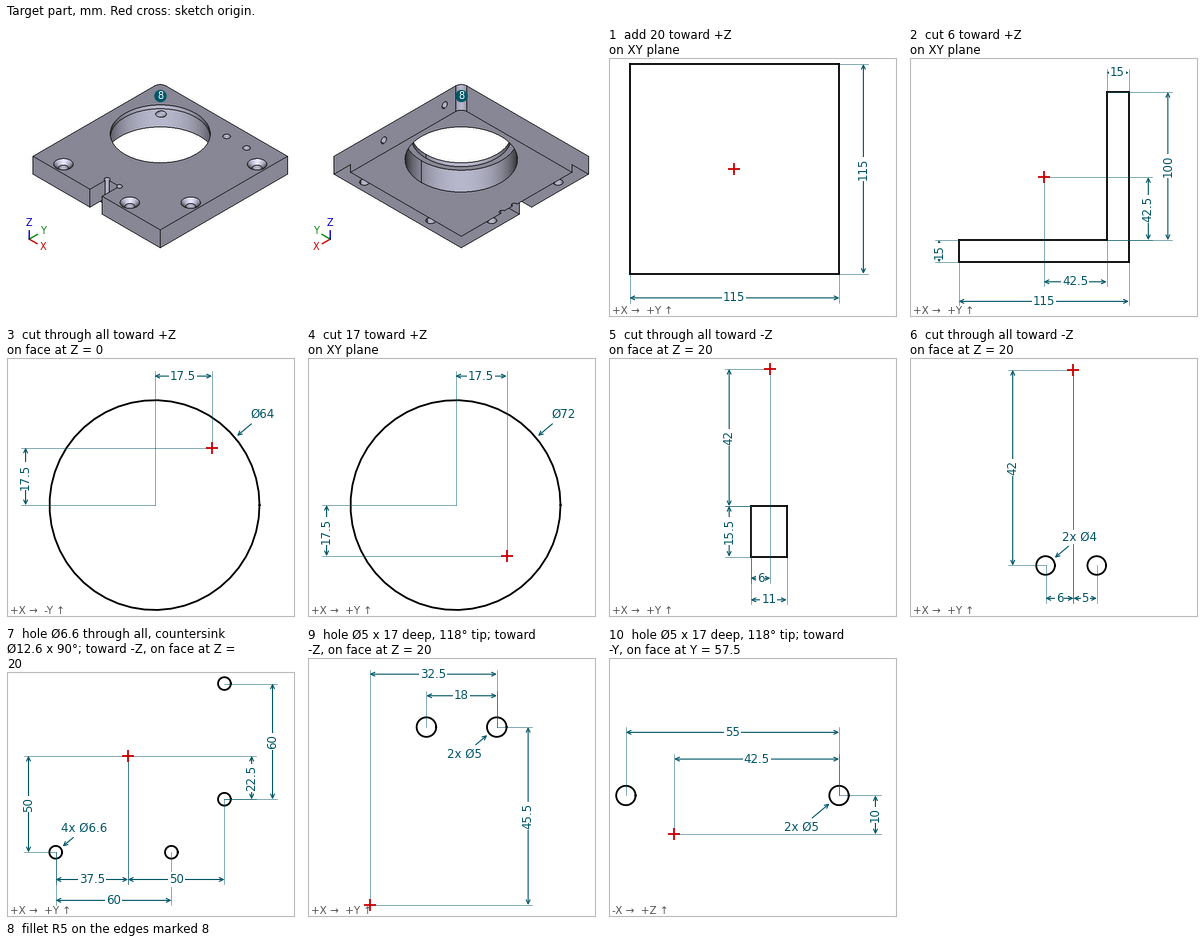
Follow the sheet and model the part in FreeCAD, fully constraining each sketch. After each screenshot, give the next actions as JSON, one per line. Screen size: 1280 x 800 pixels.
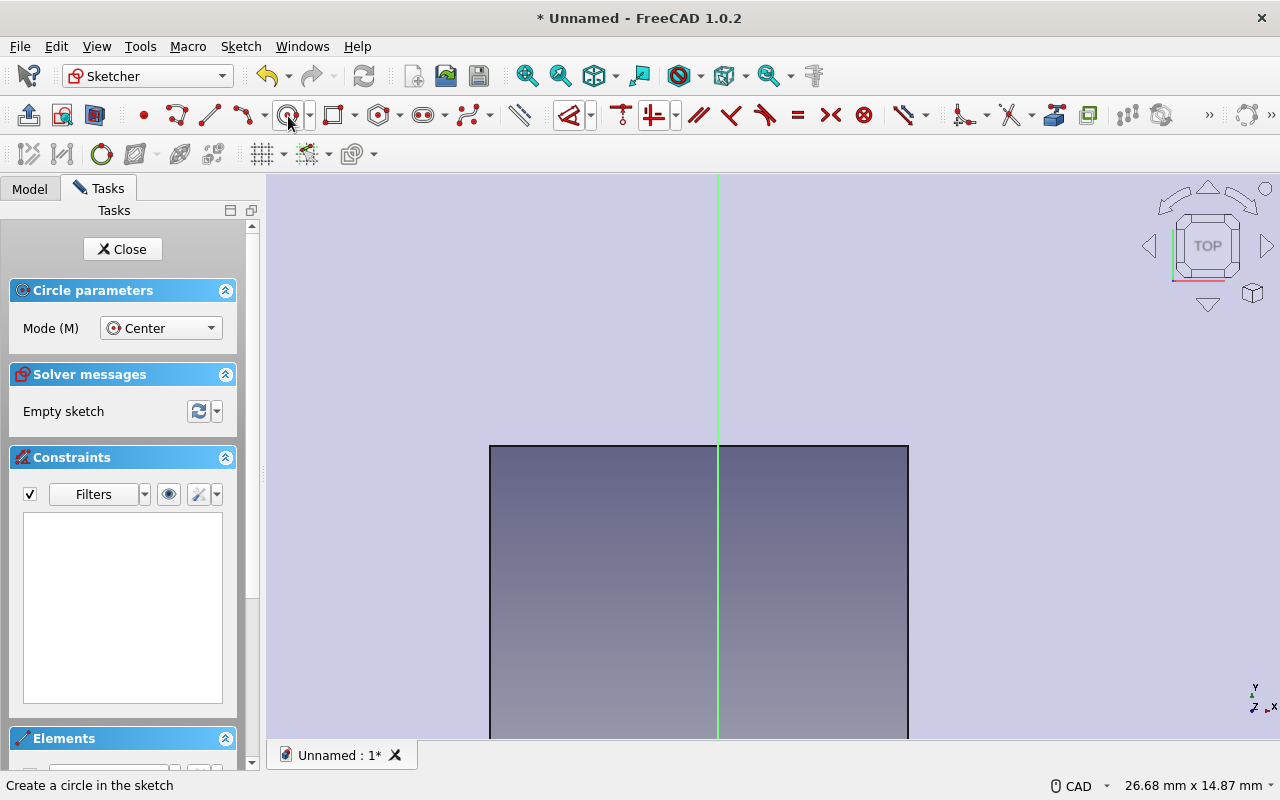
{"action": "left_click", "coordinate": [490, 446]}
{"action": "left_click", "coordinate": [544, 393]}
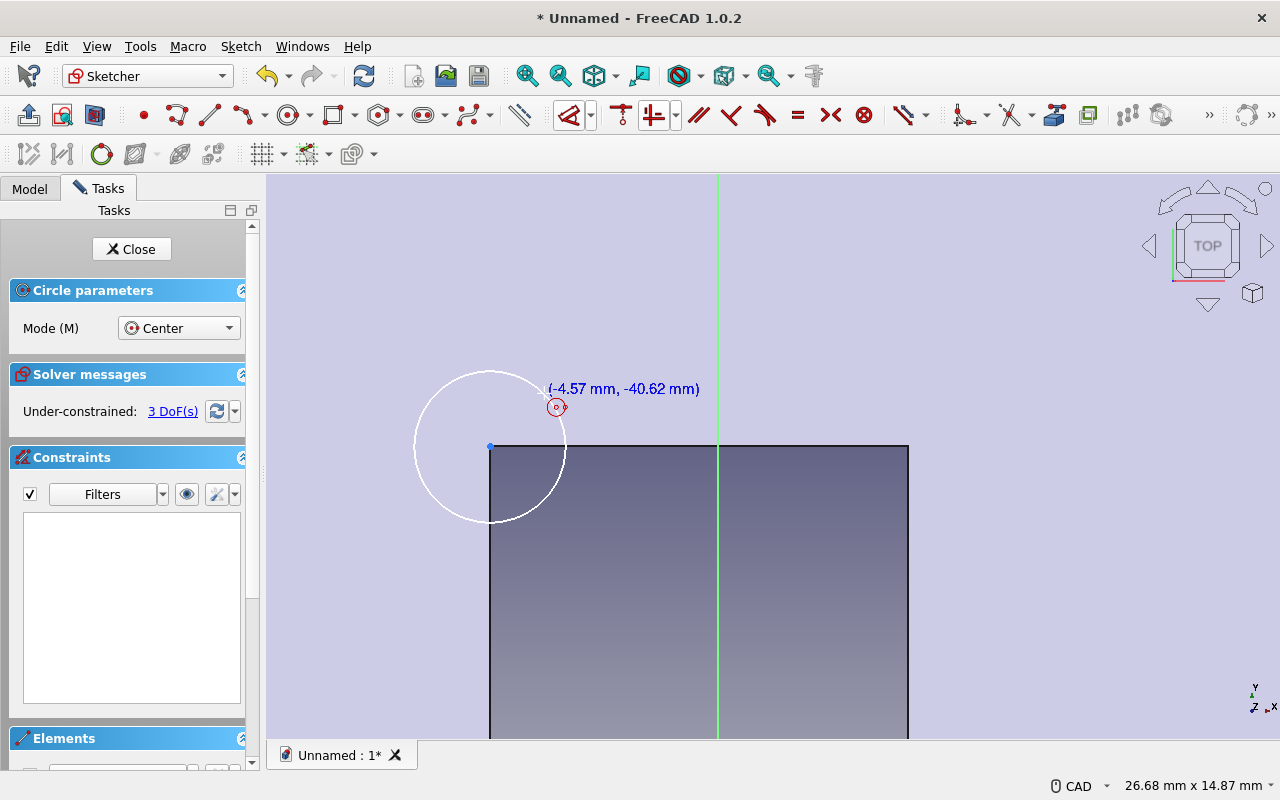
{"action": "left_click", "coordinate": [908, 446]}
{"action": "left_click", "coordinate": [962, 393]}
{"action": "key", "text": "Escape"}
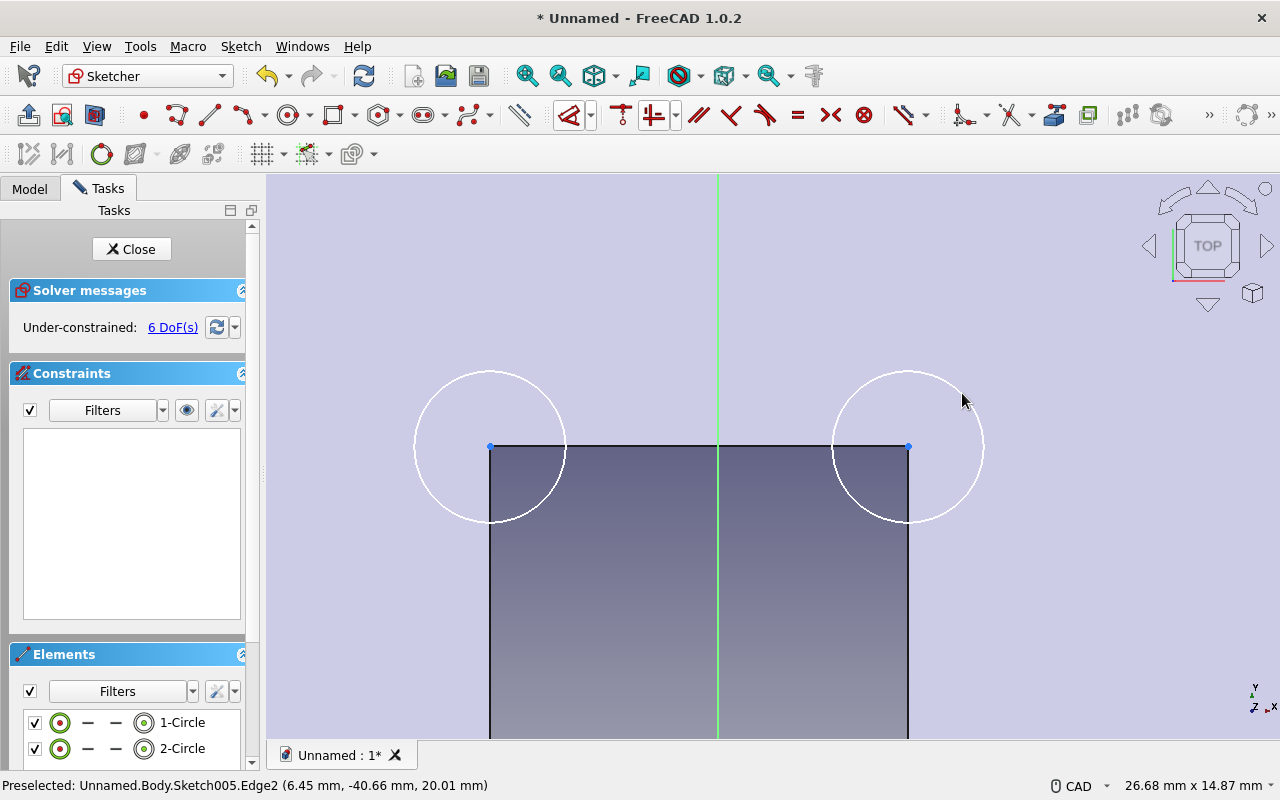
{"action": "left_click", "coordinate": [543, 393]}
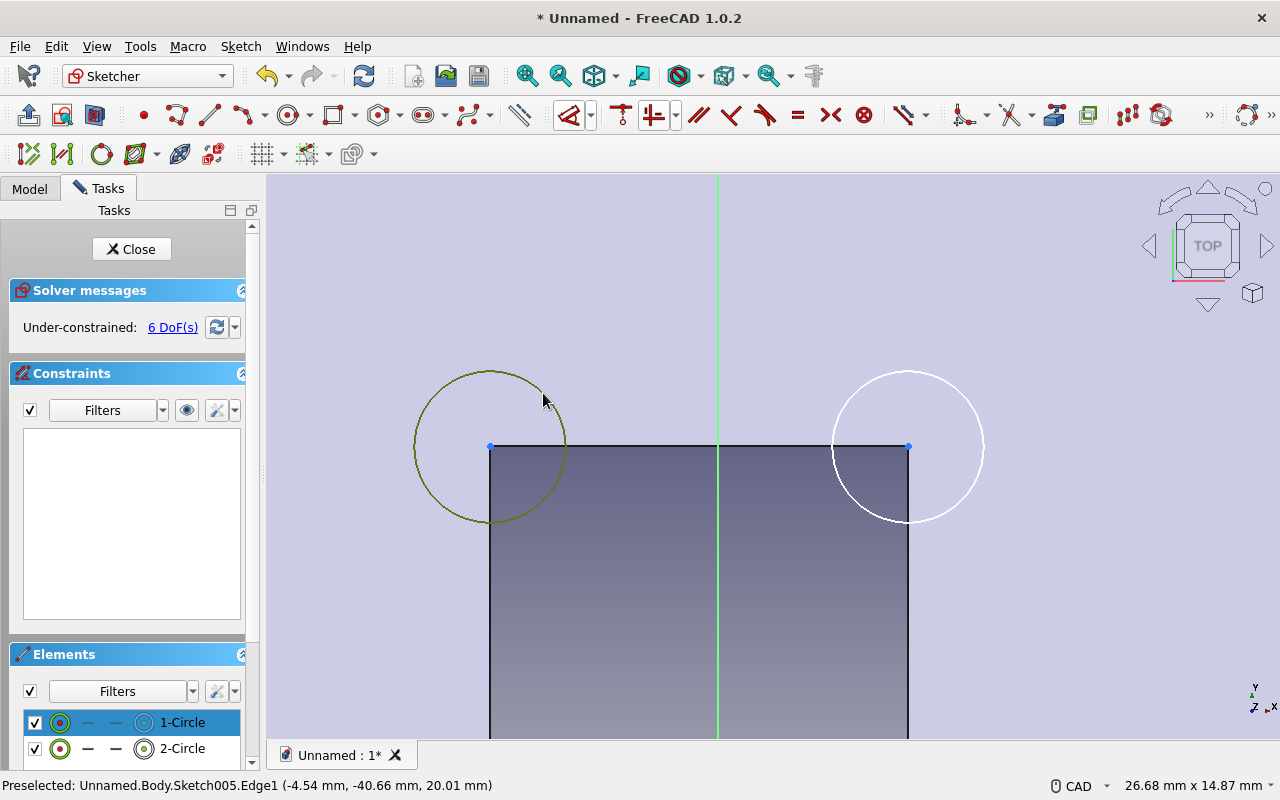
{"action": "left_click", "coordinate": [961, 393]}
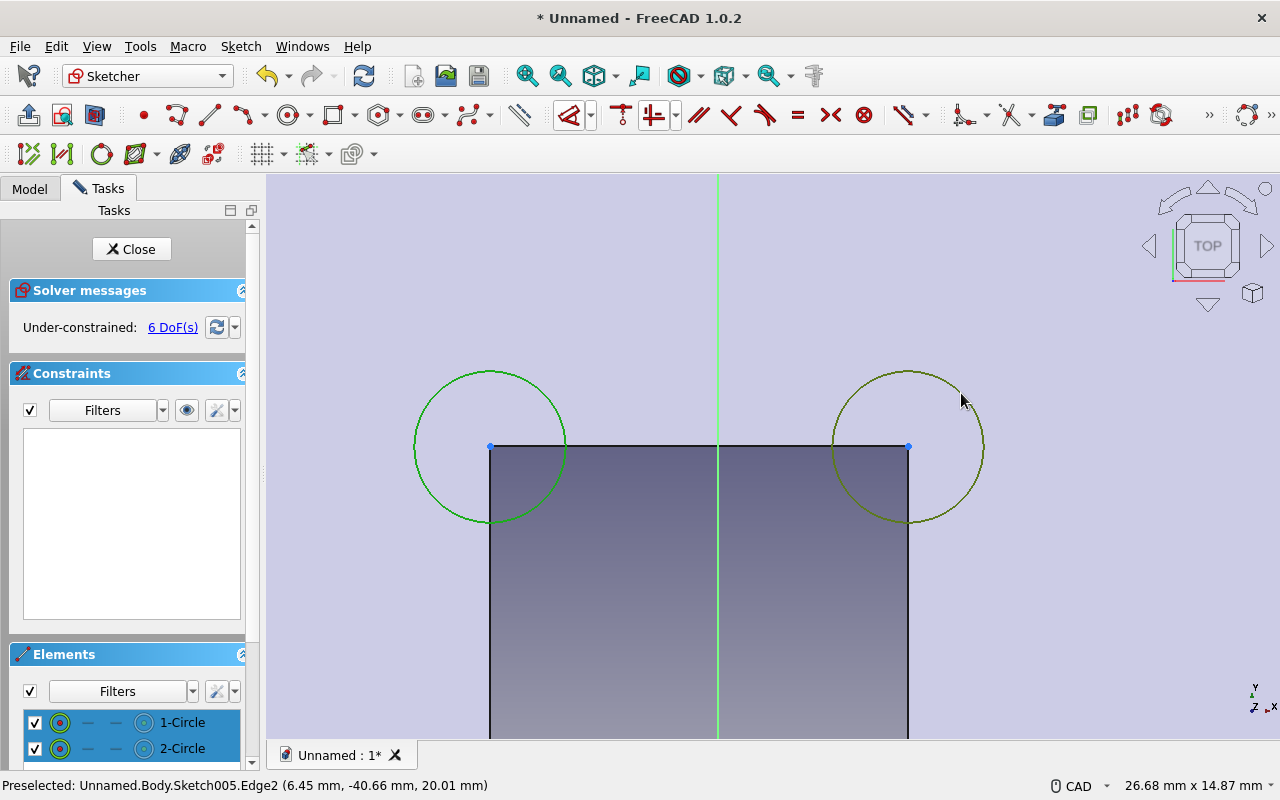
{"action": "key", "text": "e"}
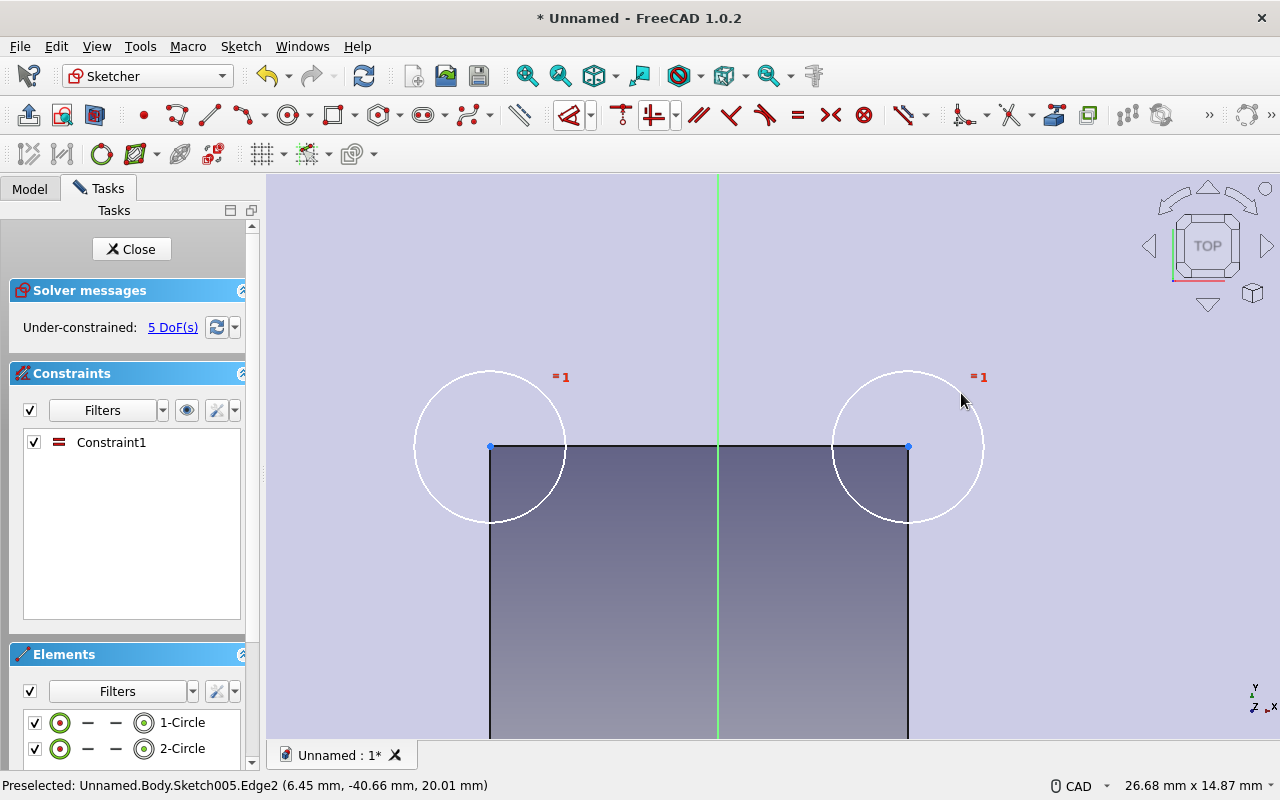
{"action": "left_click", "coordinate": [490, 447]}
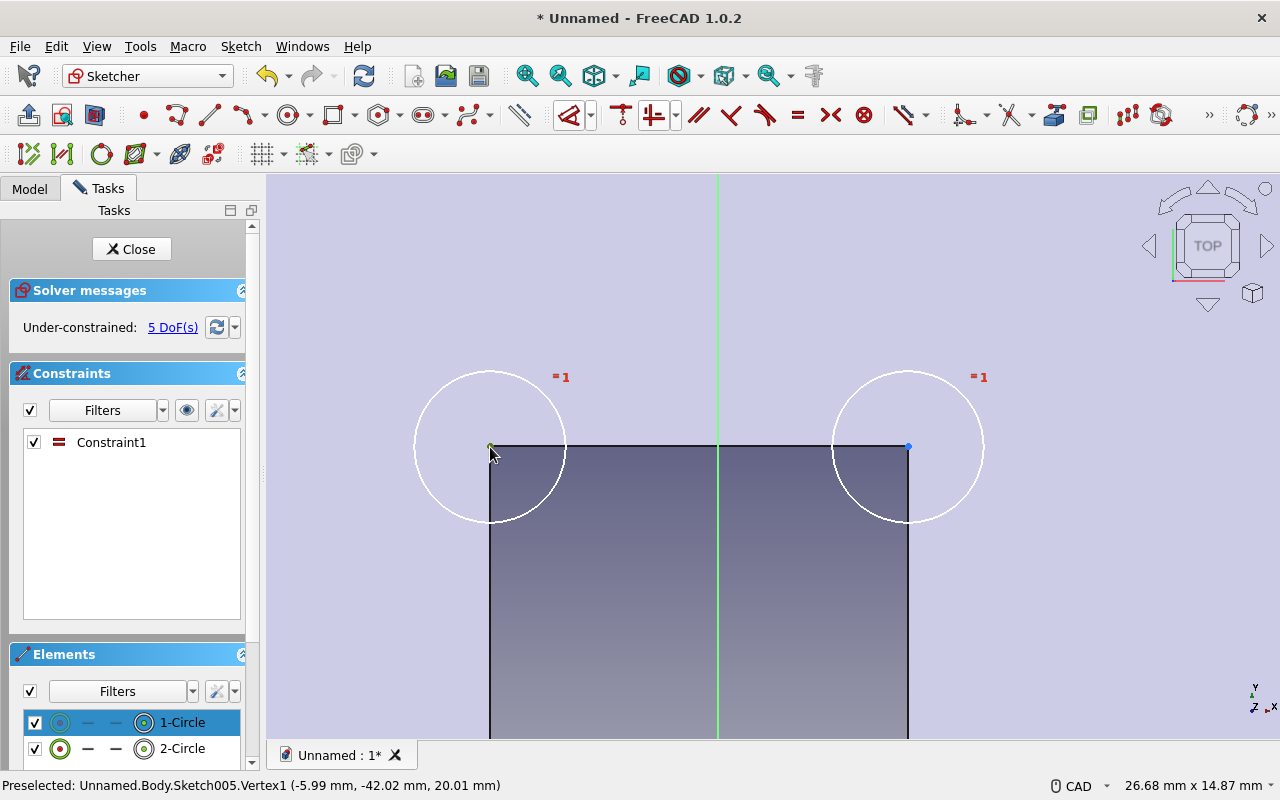
{"action": "left_click", "coordinate": [908, 447]}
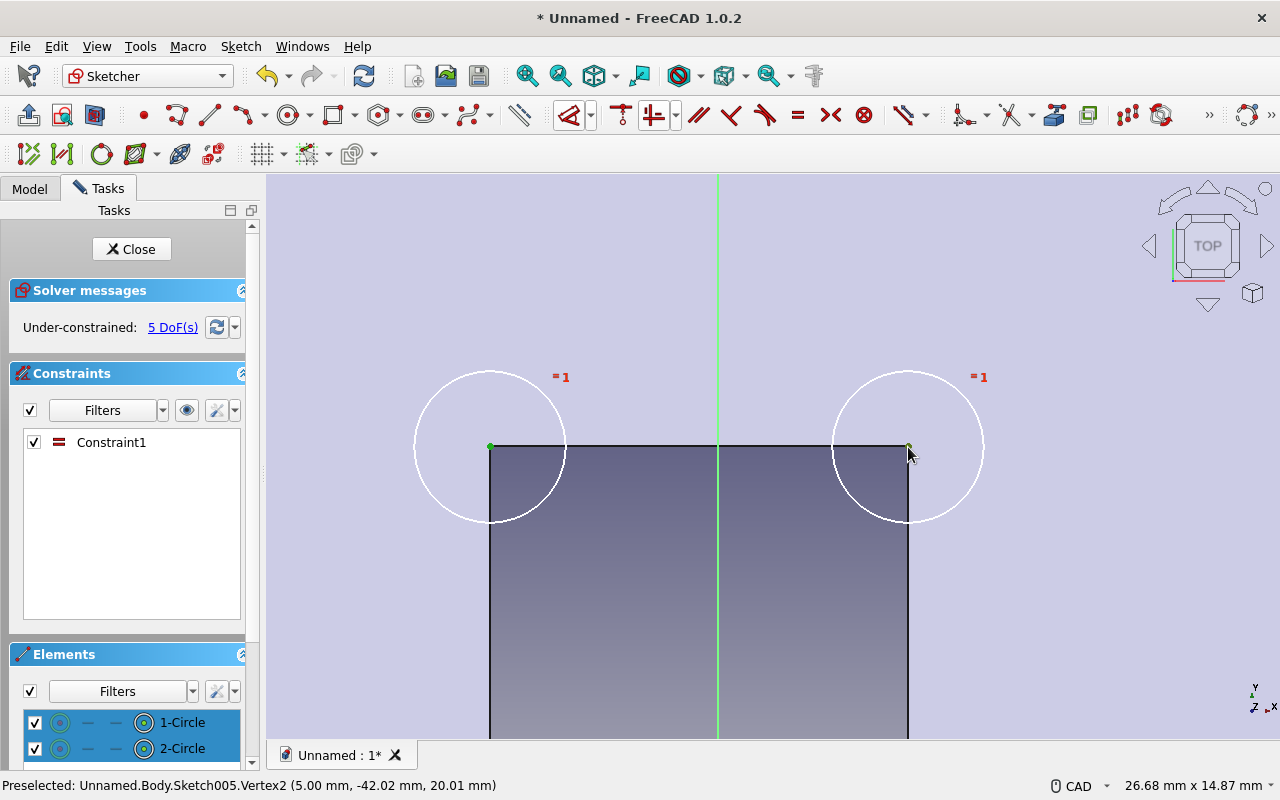
{"action": "key", "text": "h"}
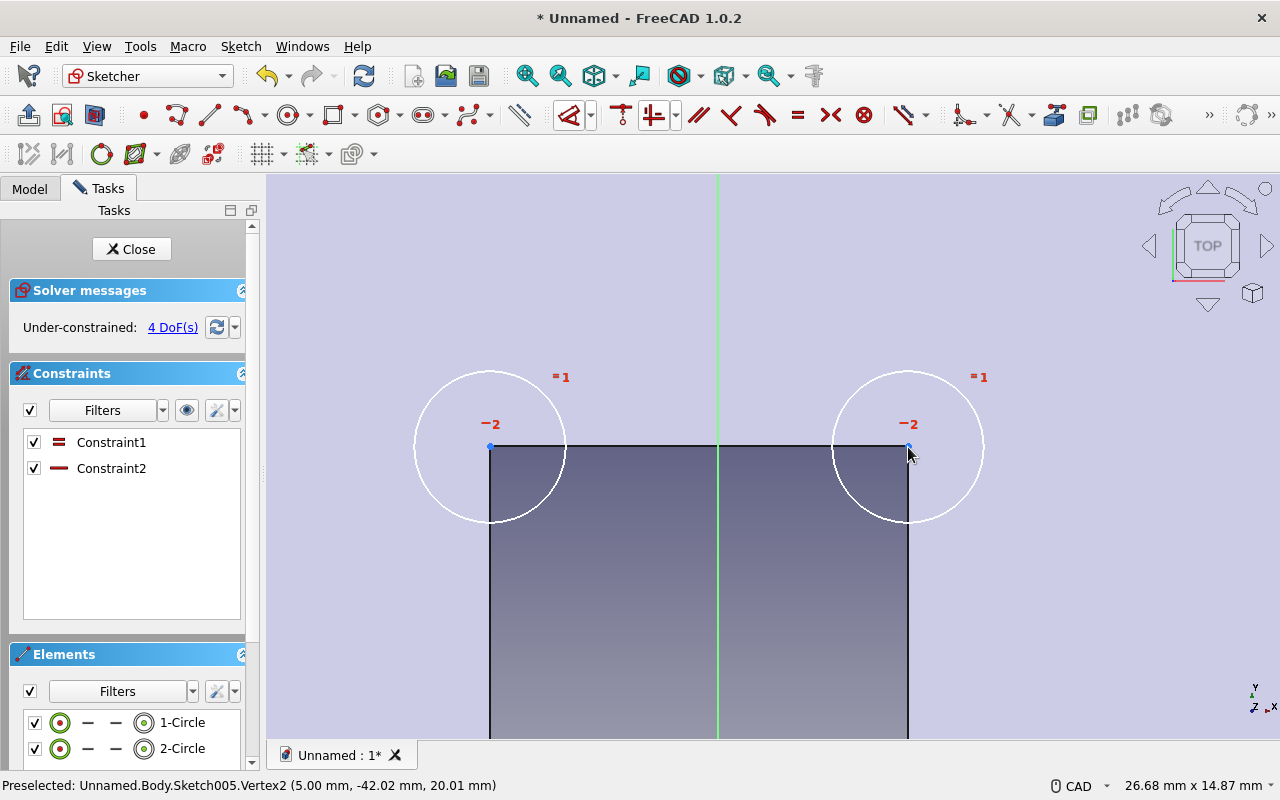
{"action": "left_click", "coordinate": [543, 393]}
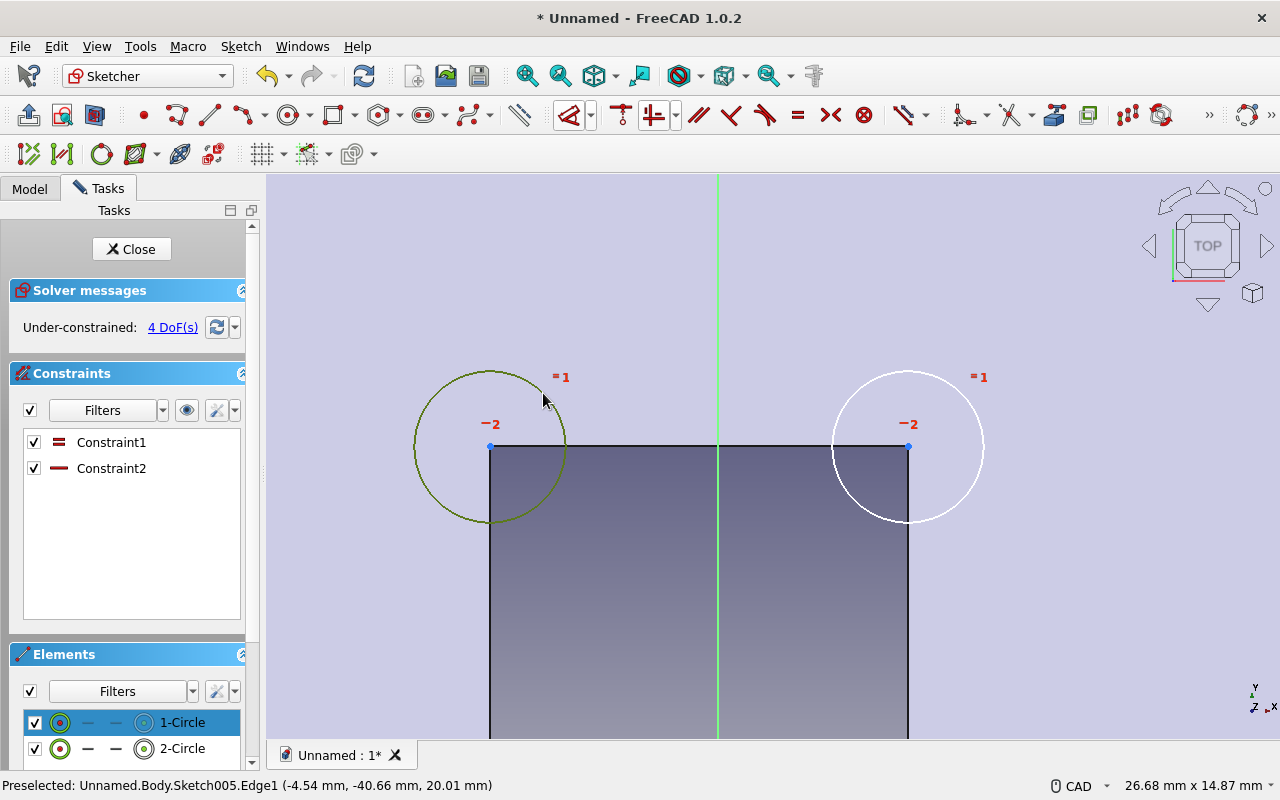
{"action": "left_click", "coordinate": [590, 116]}